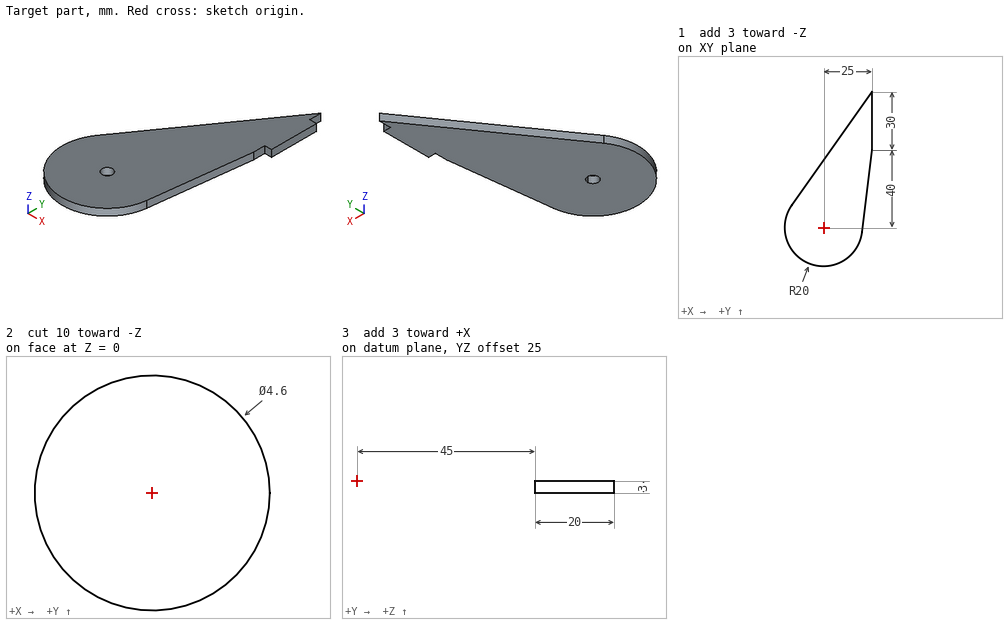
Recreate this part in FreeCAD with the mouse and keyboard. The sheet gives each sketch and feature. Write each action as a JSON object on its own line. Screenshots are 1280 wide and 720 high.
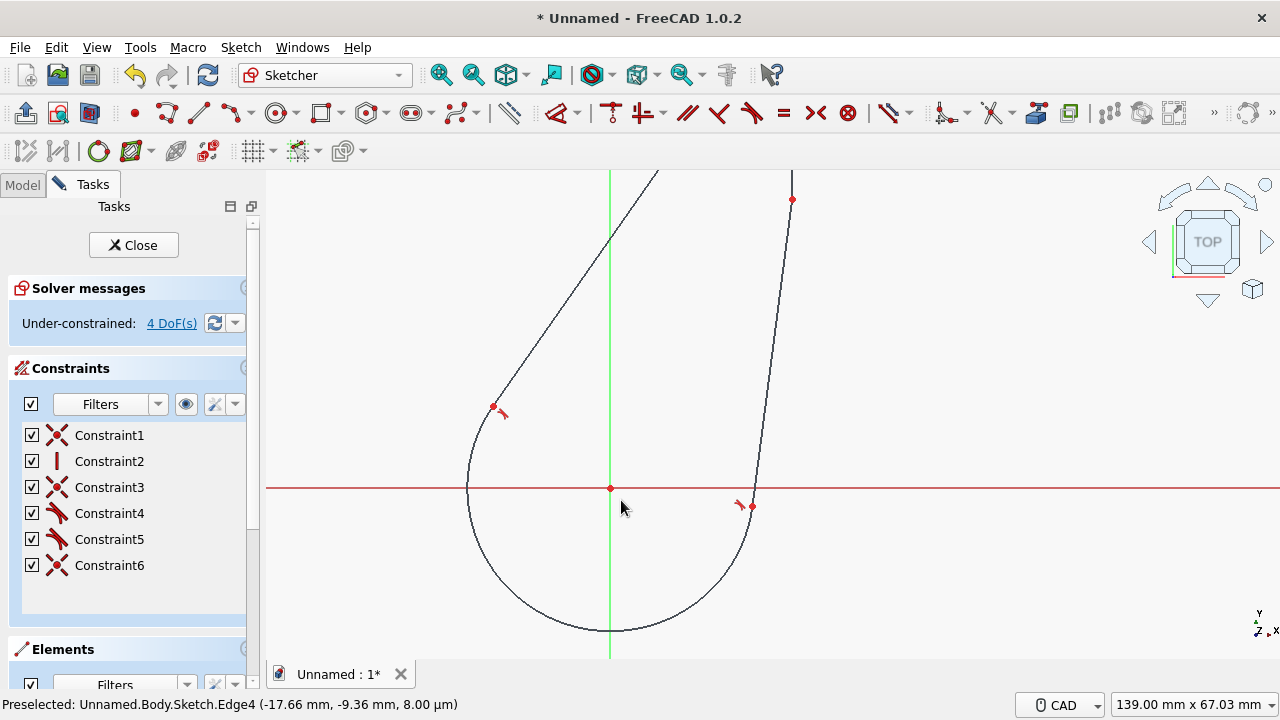
{"action": "left_click", "coordinate": [483, 554]}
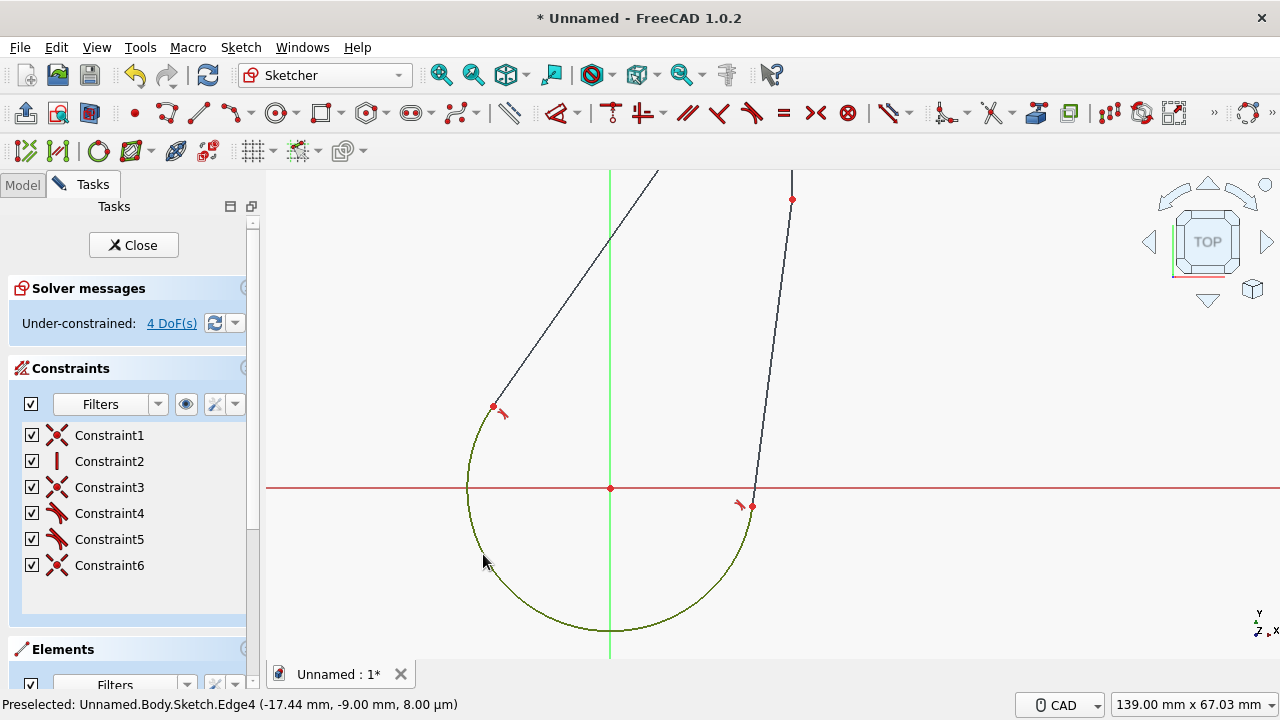
{"action": "key", "text": "k r"}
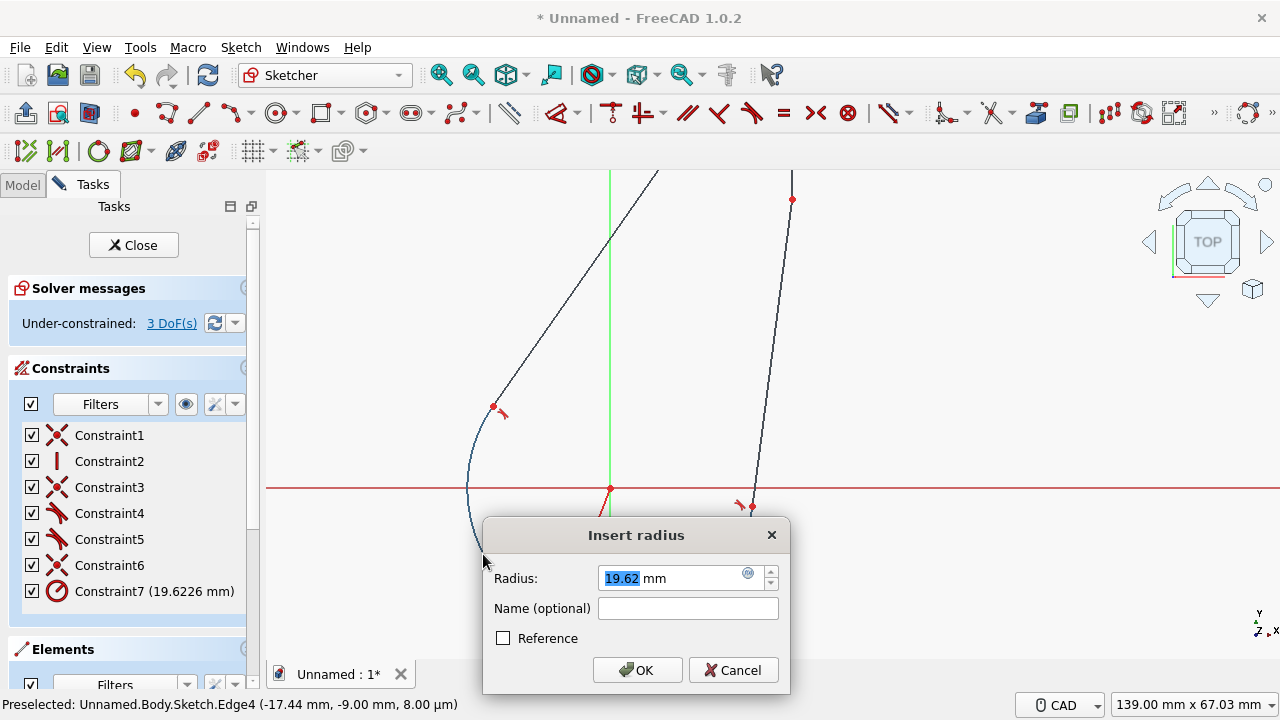
{"action": "type", "text": "20"}
{"action": "key", "text": "Return"}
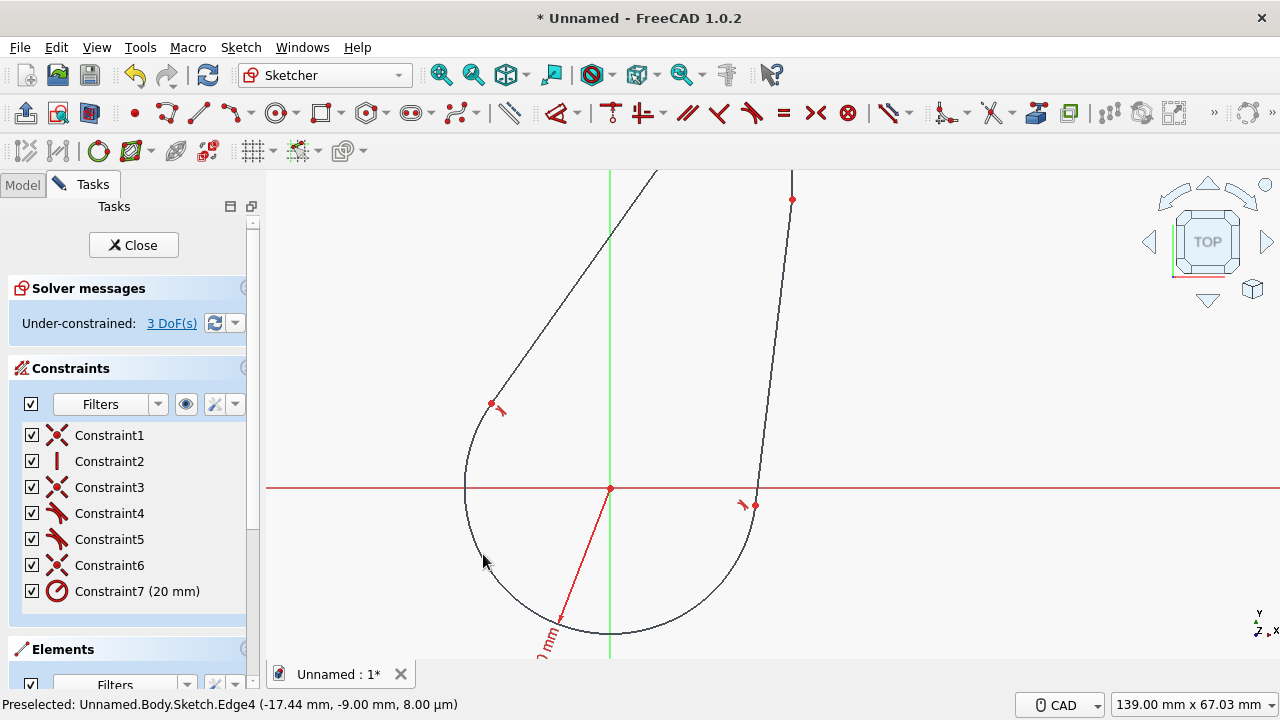
{"action": "scroll", "coordinate": [755, 507], "scroll_direction": "down", "scroll_amount": 4}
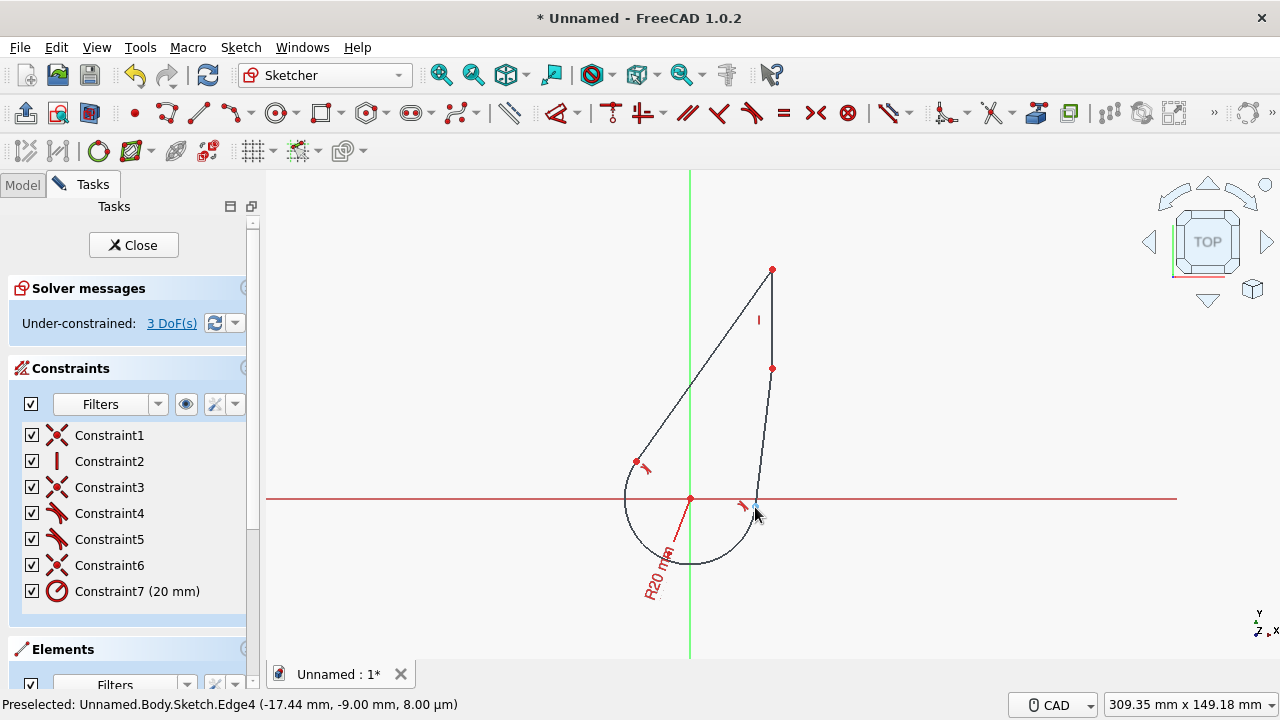
{"action": "left_click", "coordinate": [772, 339]}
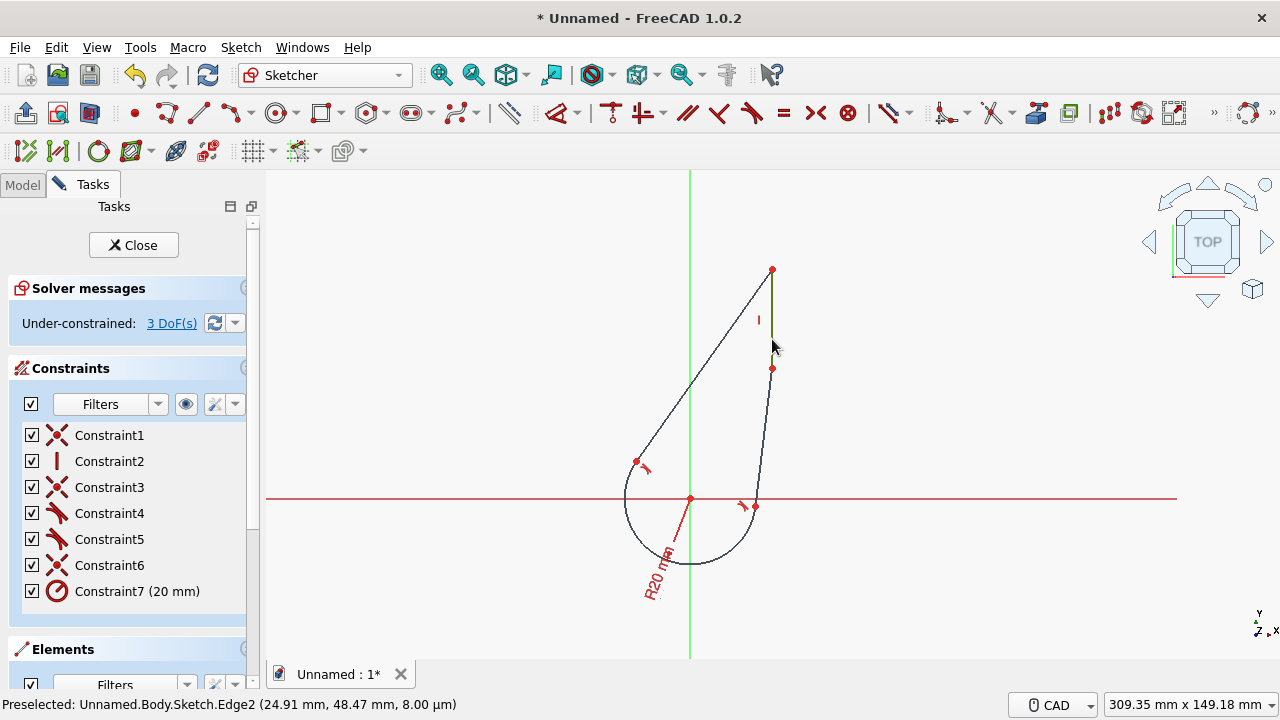
{"action": "left_click", "coordinate": [580, 114]}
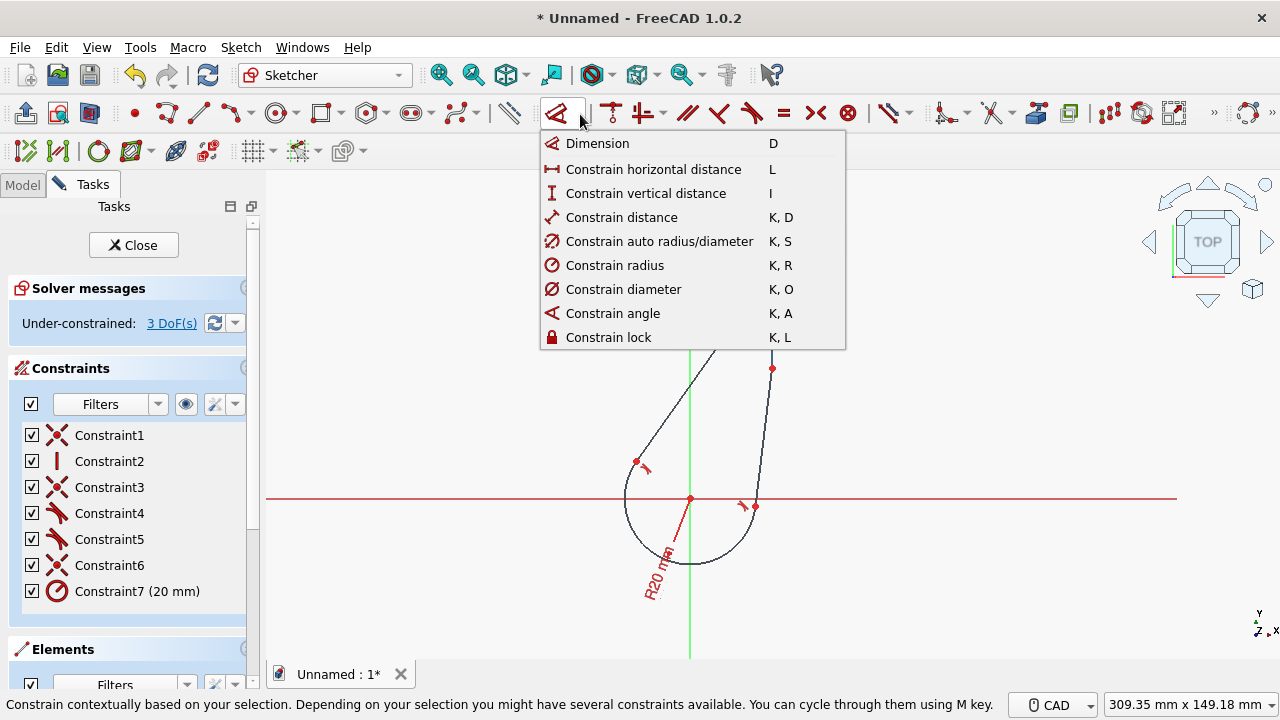
{"action": "left_click", "coordinate": [693, 193]}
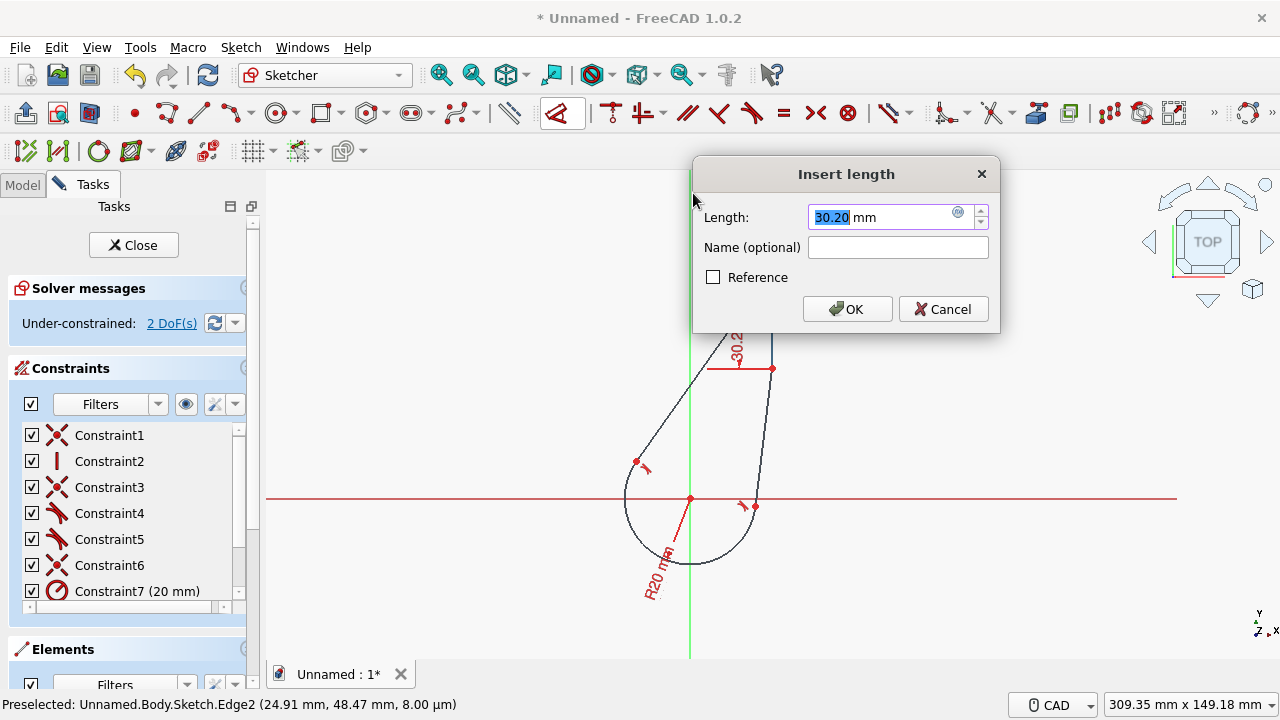
{"action": "type", "text": "30"}
{"action": "key", "text": "Return"}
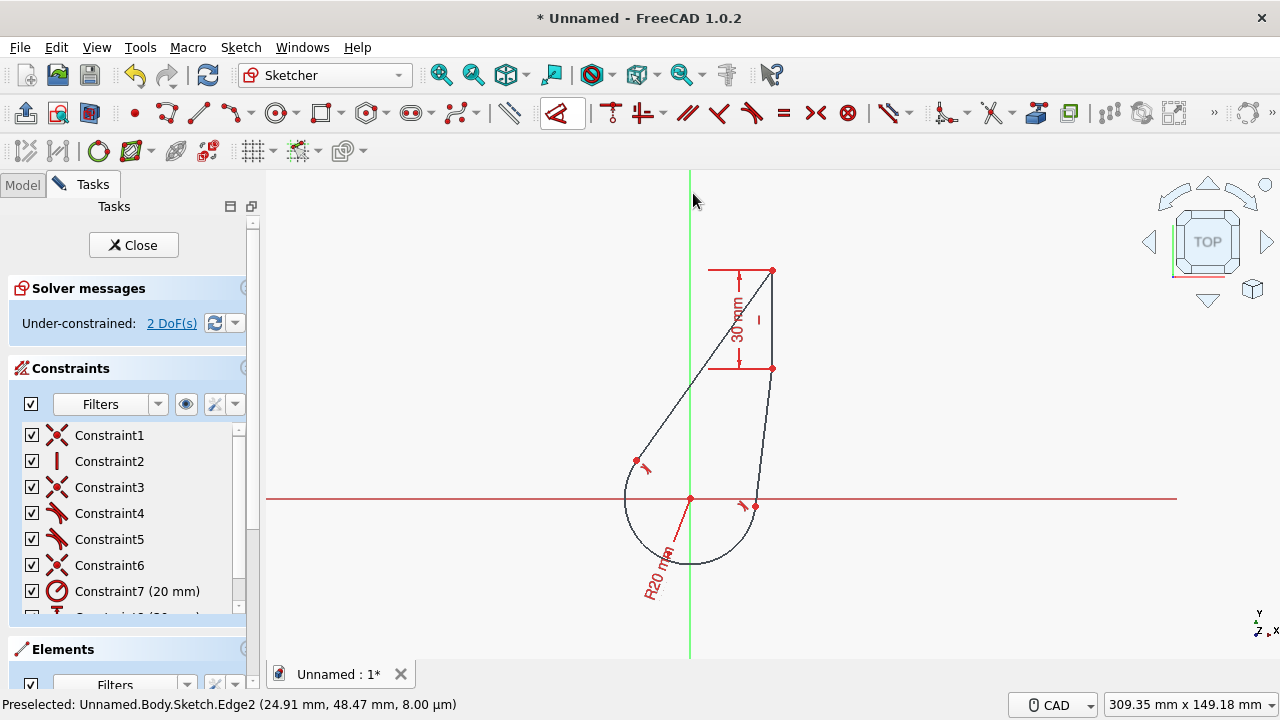
{"action": "left_click", "coordinate": [772, 369]}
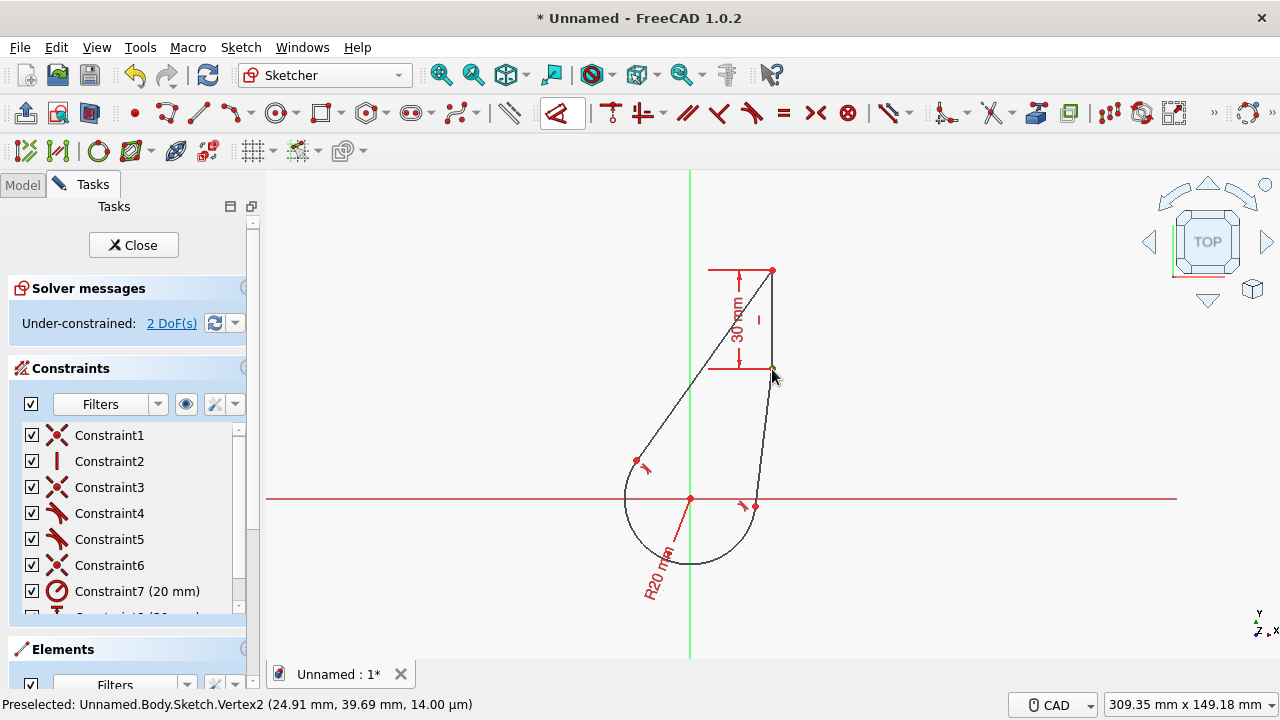
{"action": "key", "text": "l"}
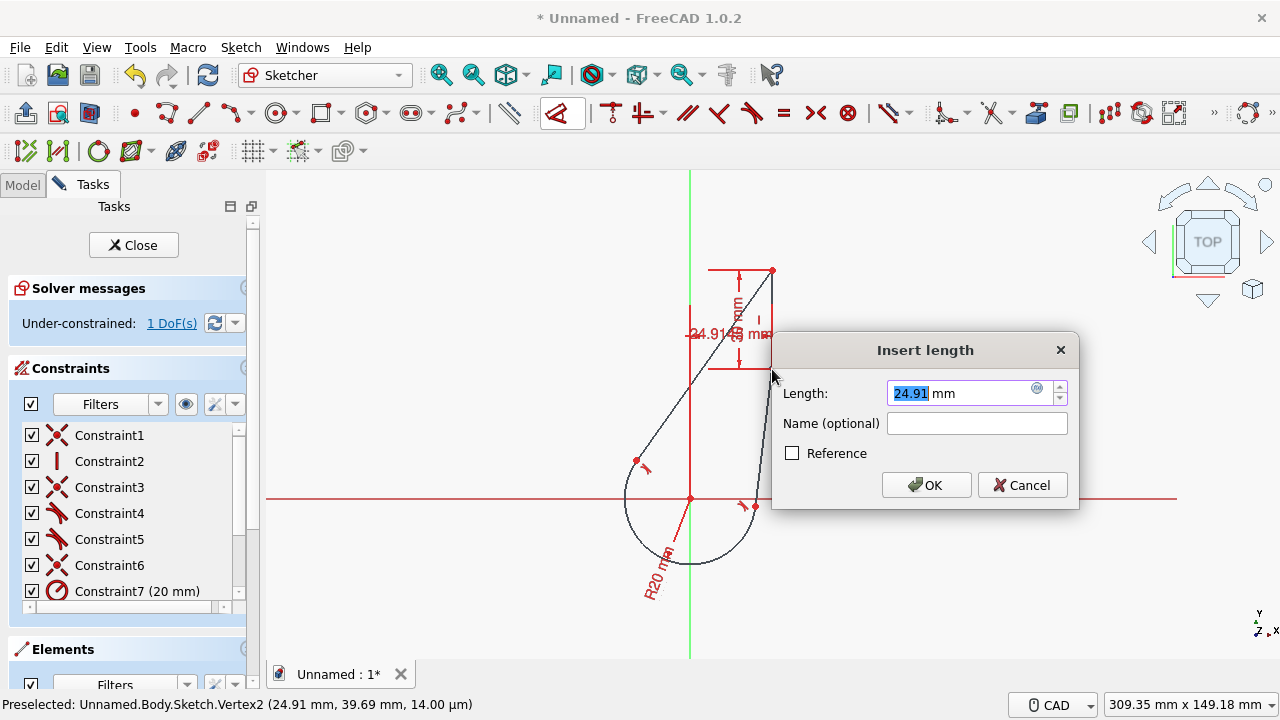
{"action": "type", "text": "25"}
{"action": "key", "text": "Return"}